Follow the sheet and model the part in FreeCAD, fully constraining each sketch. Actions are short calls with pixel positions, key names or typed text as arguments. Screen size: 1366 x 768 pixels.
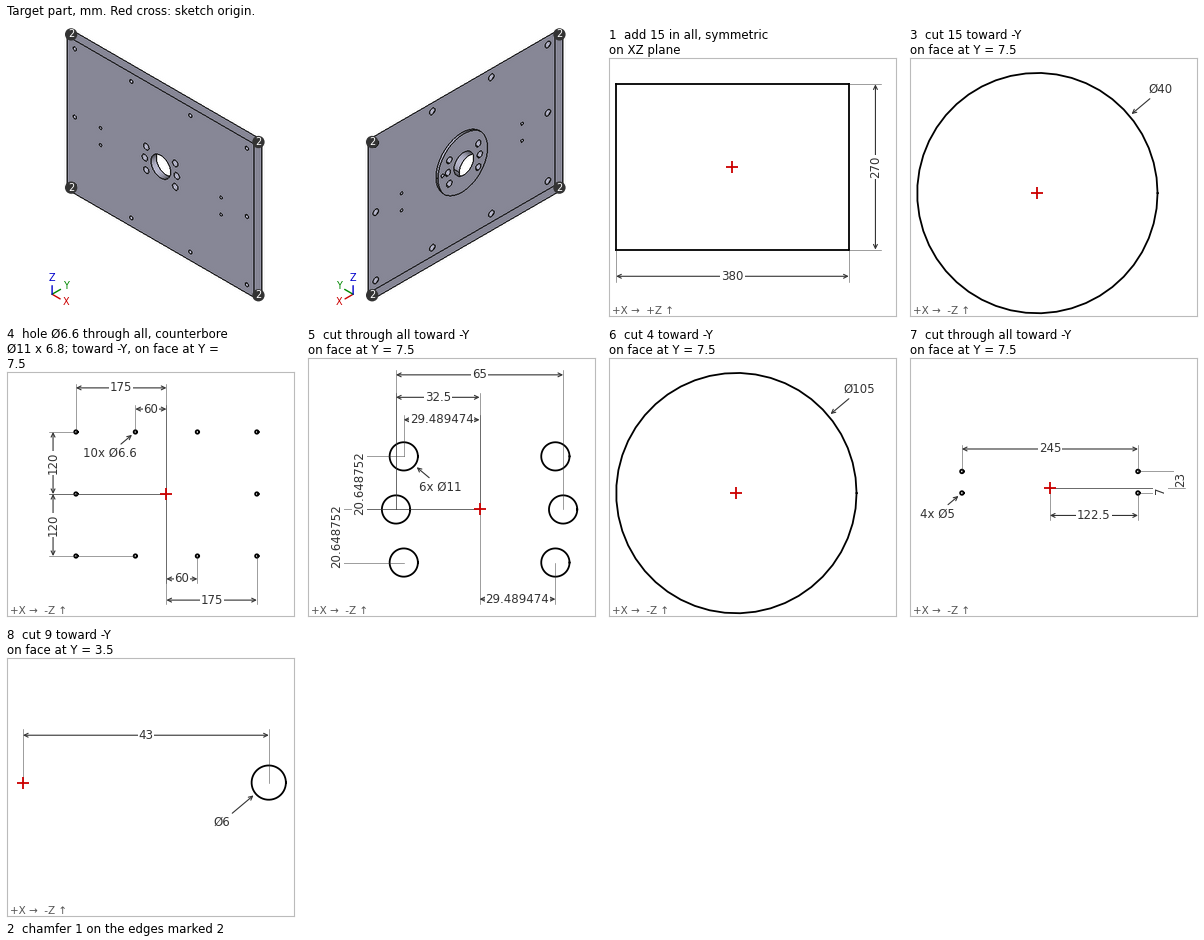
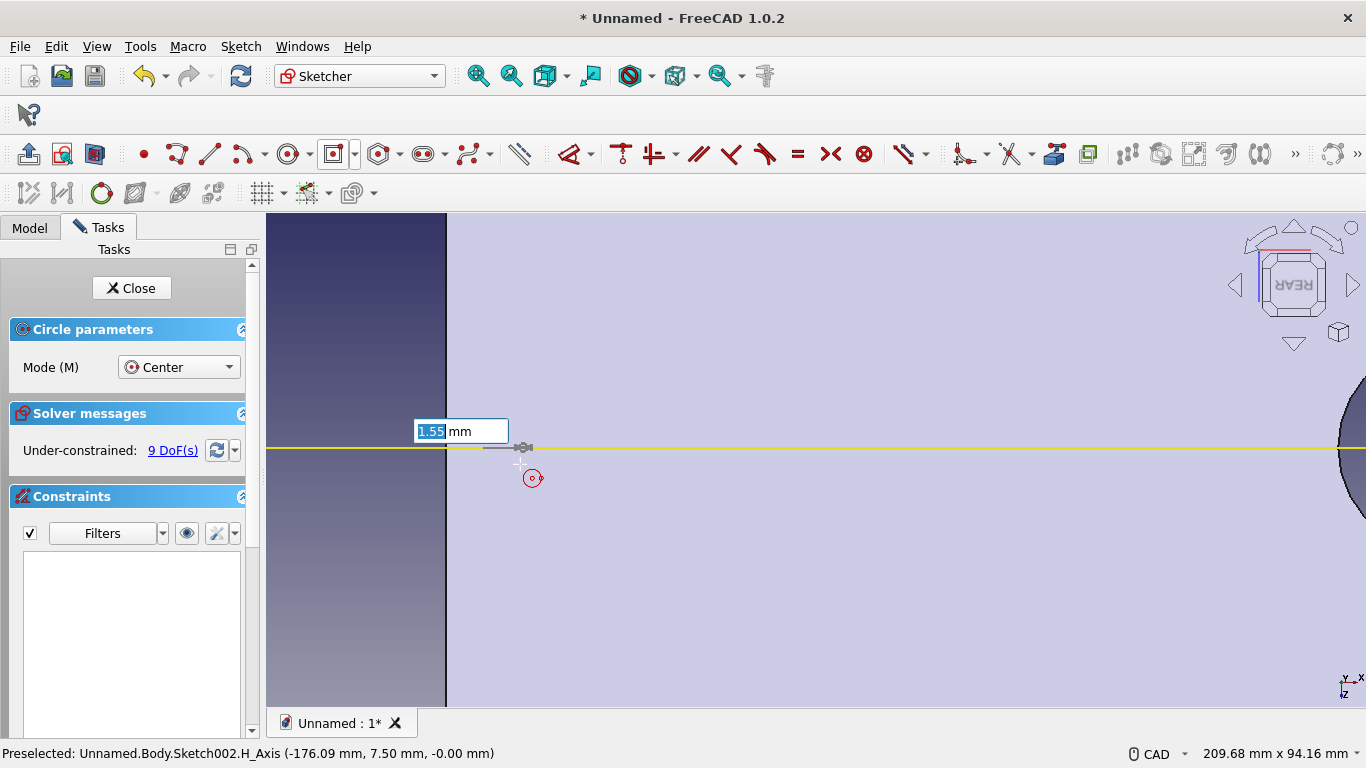
click(519, 464)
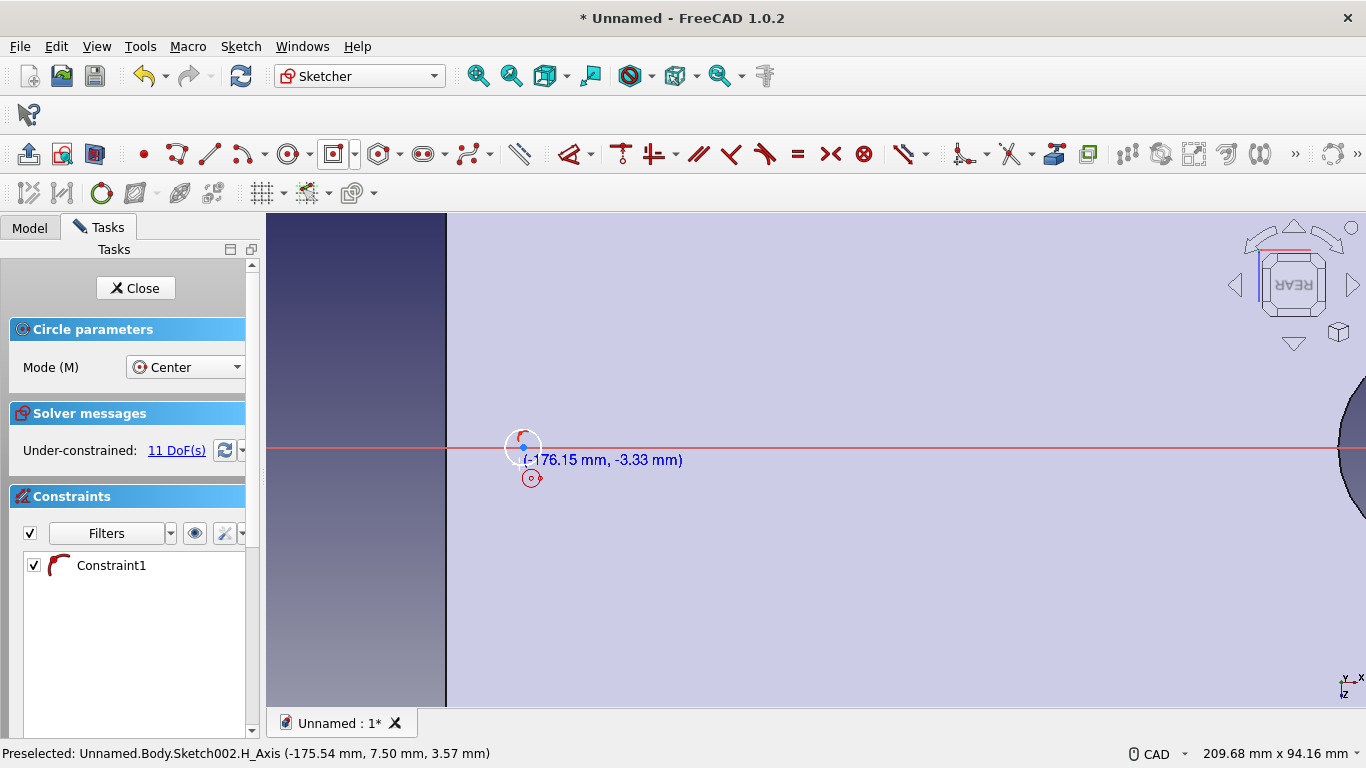
scroll(520, 464, down, 7)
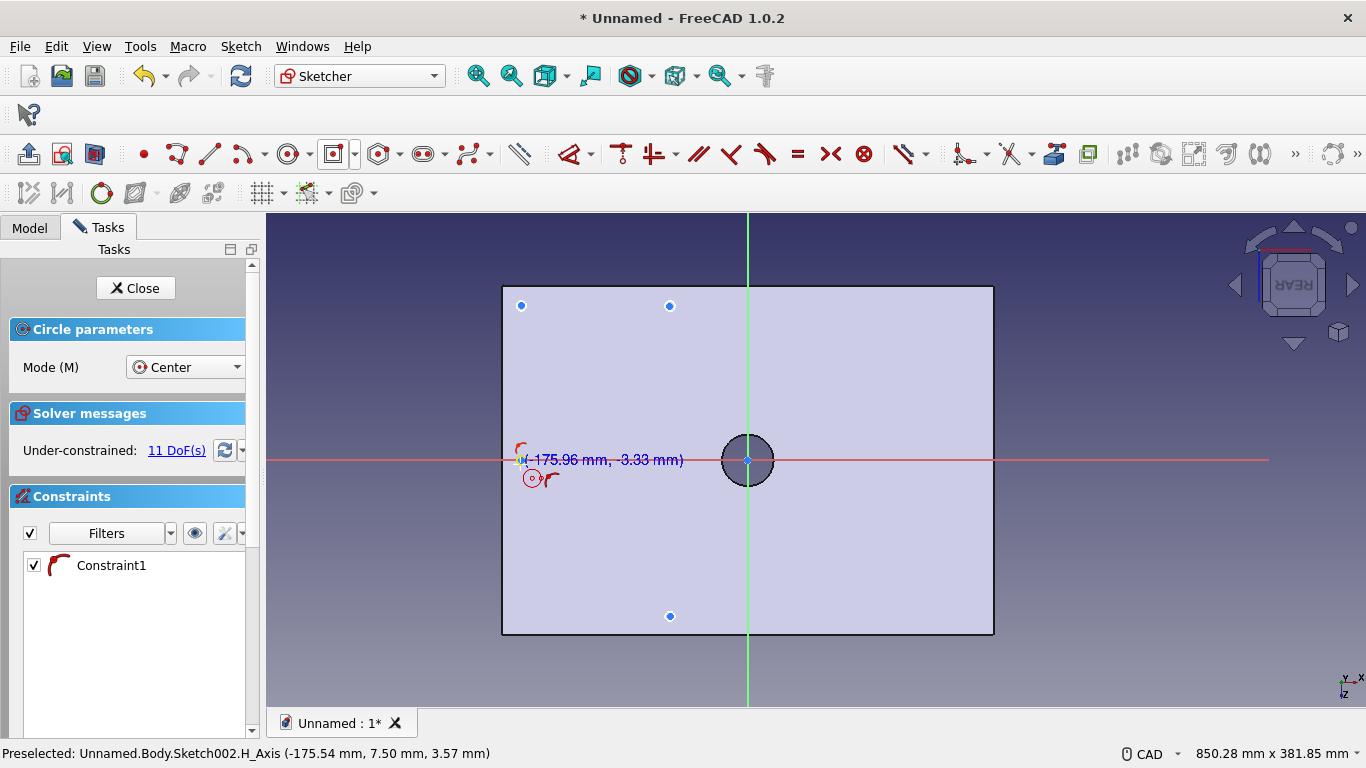
scroll(521, 616, up, 9)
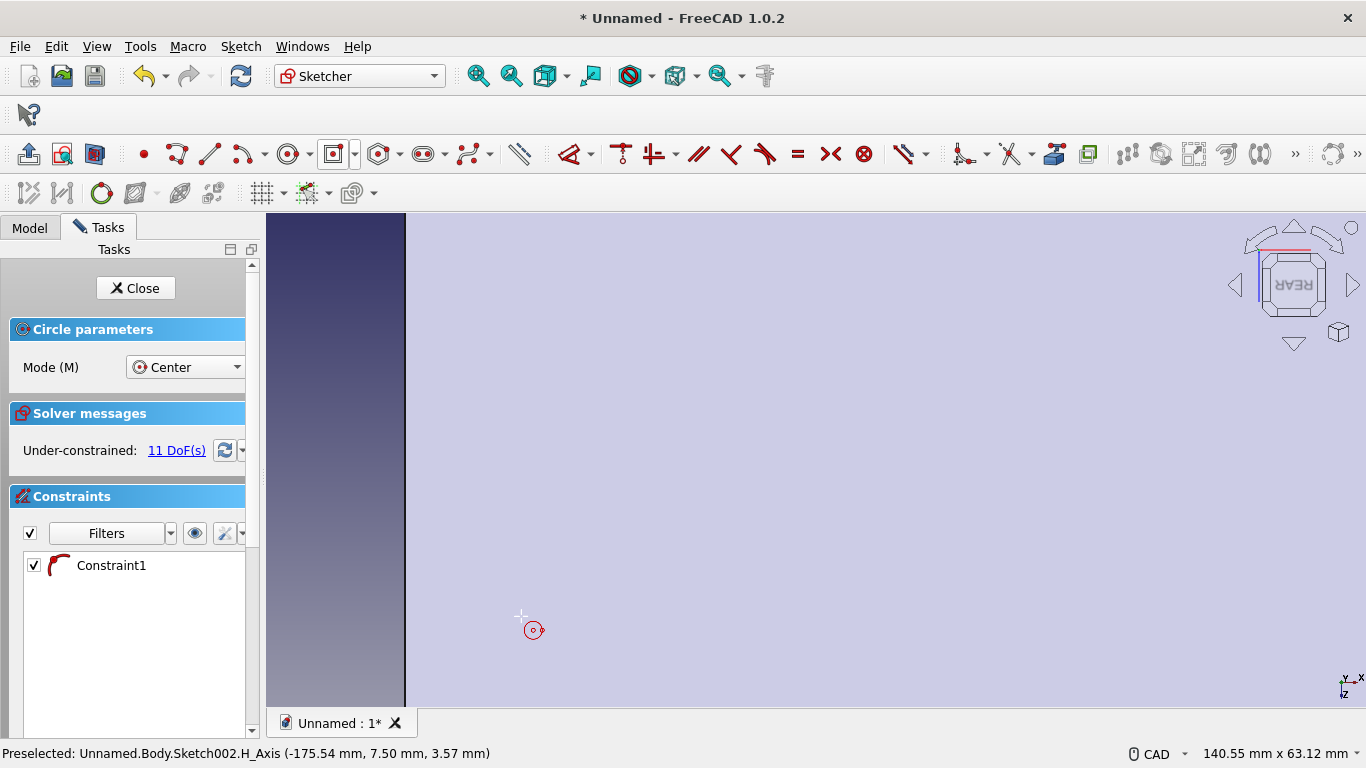
scroll(521, 616, down, 9)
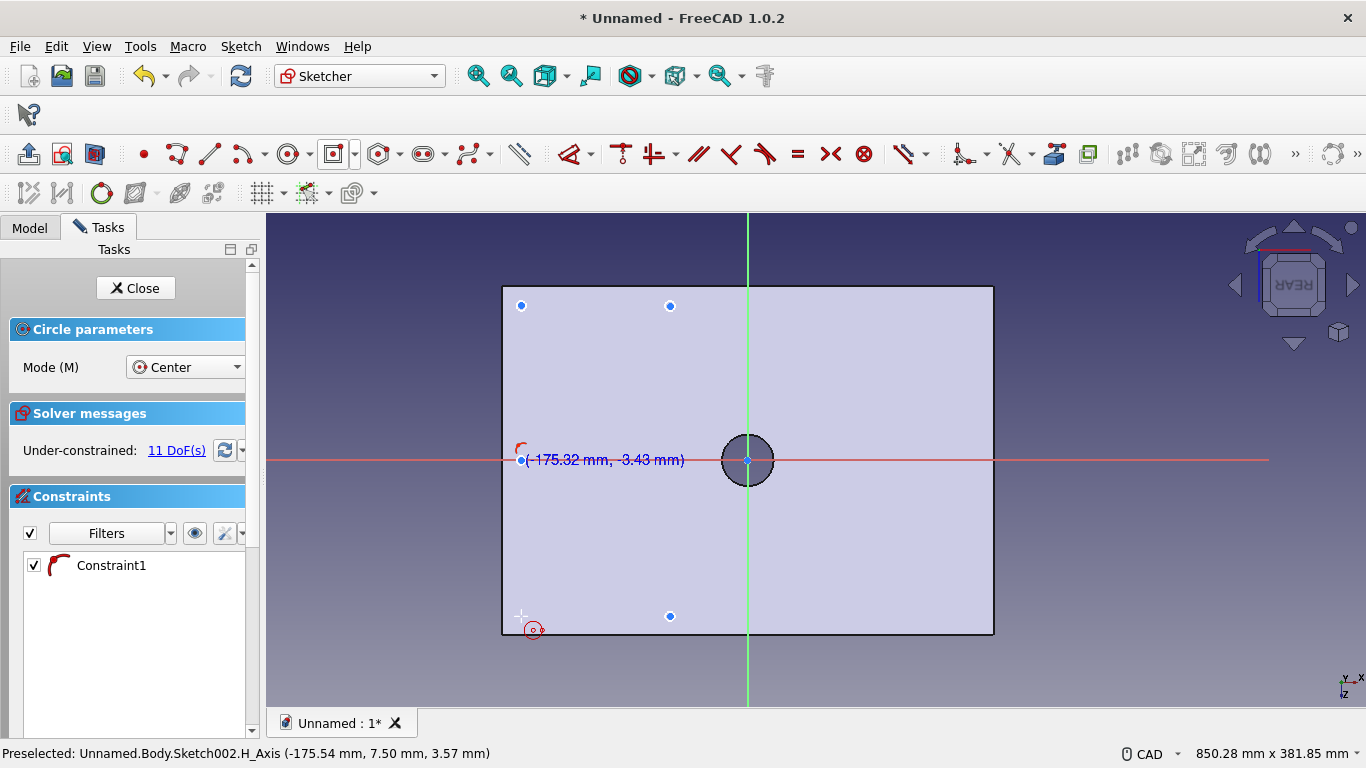
click(521, 616)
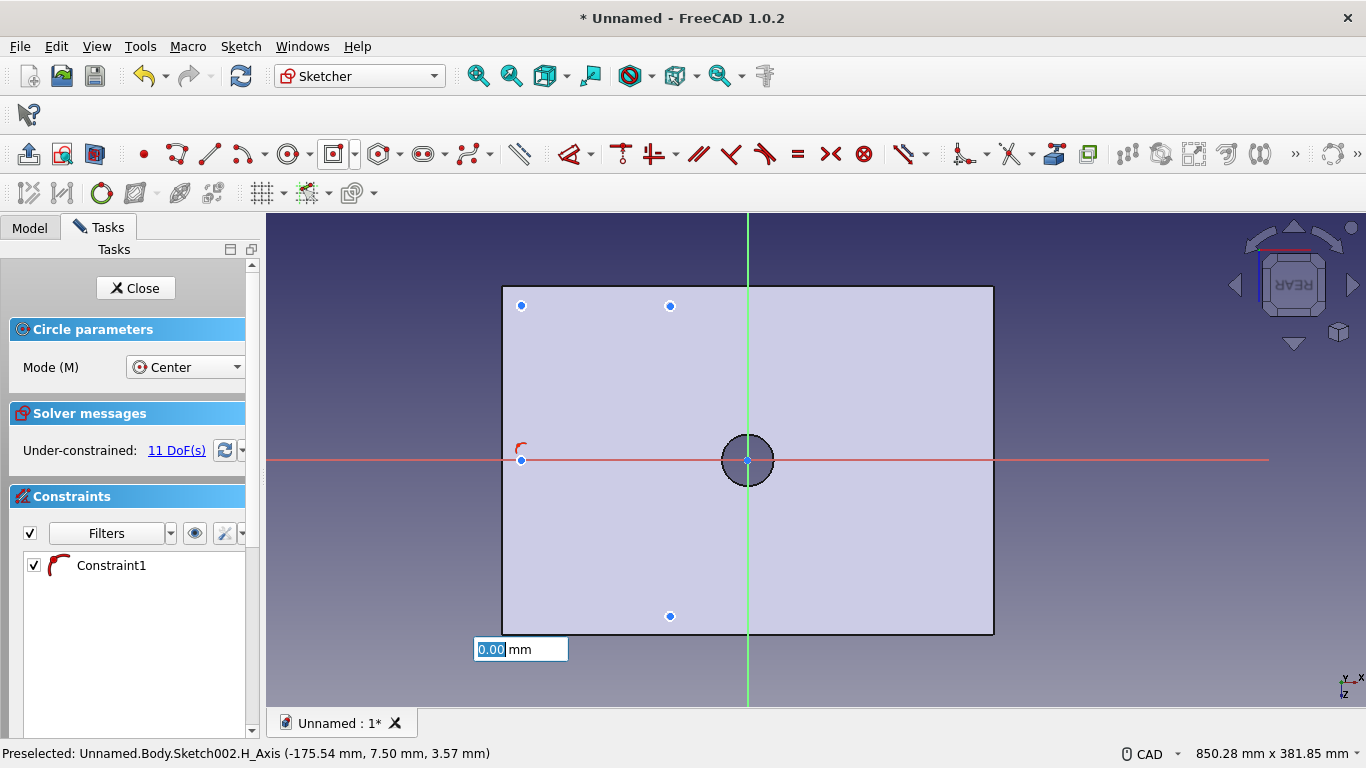
scroll(524, 613, up, 7)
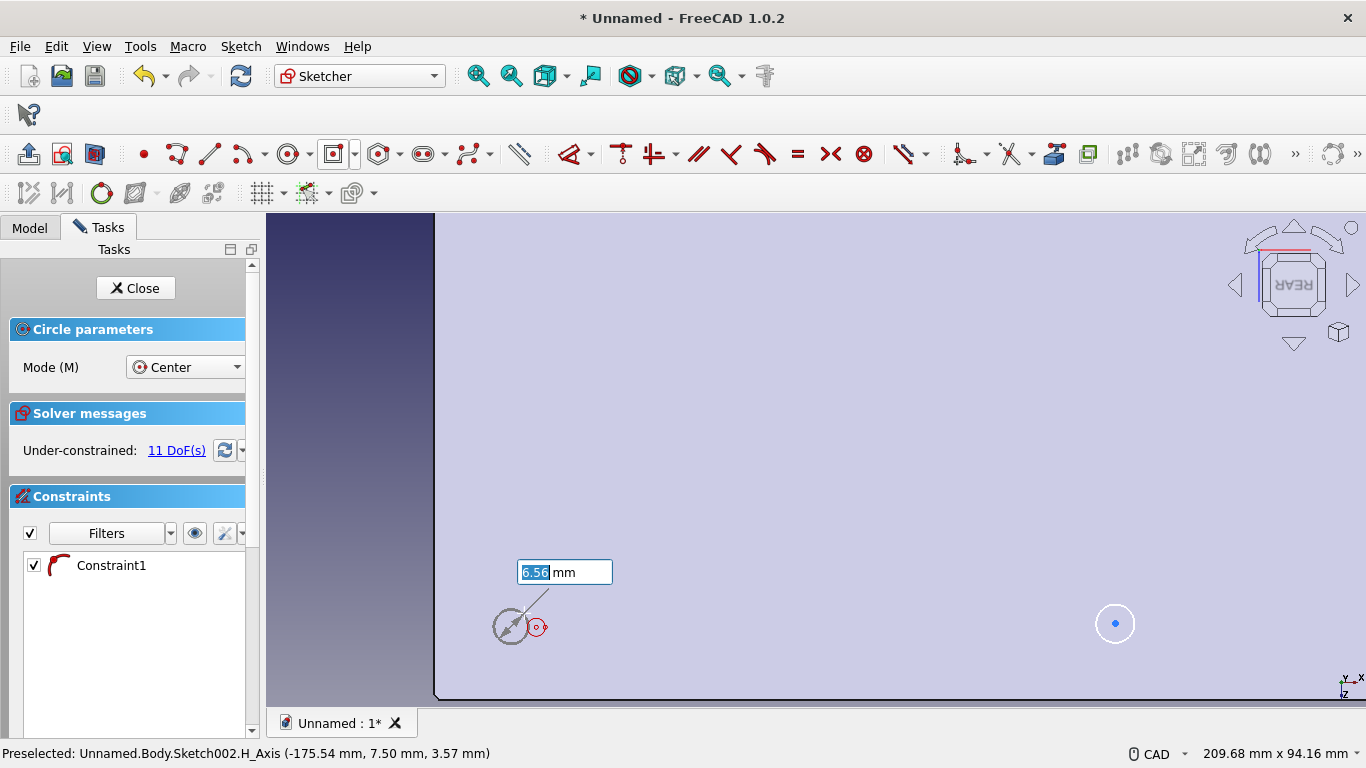
click(525, 609)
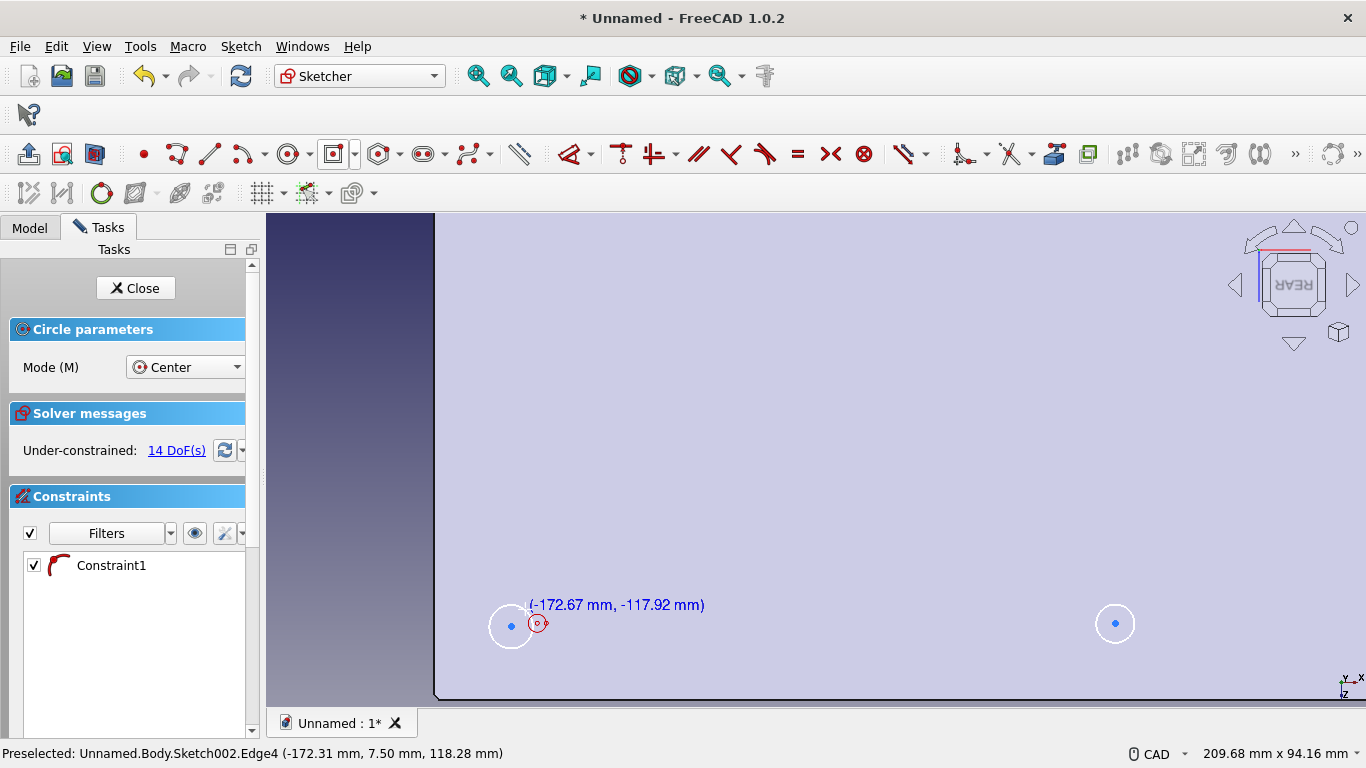
scroll(524, 613, down, 7)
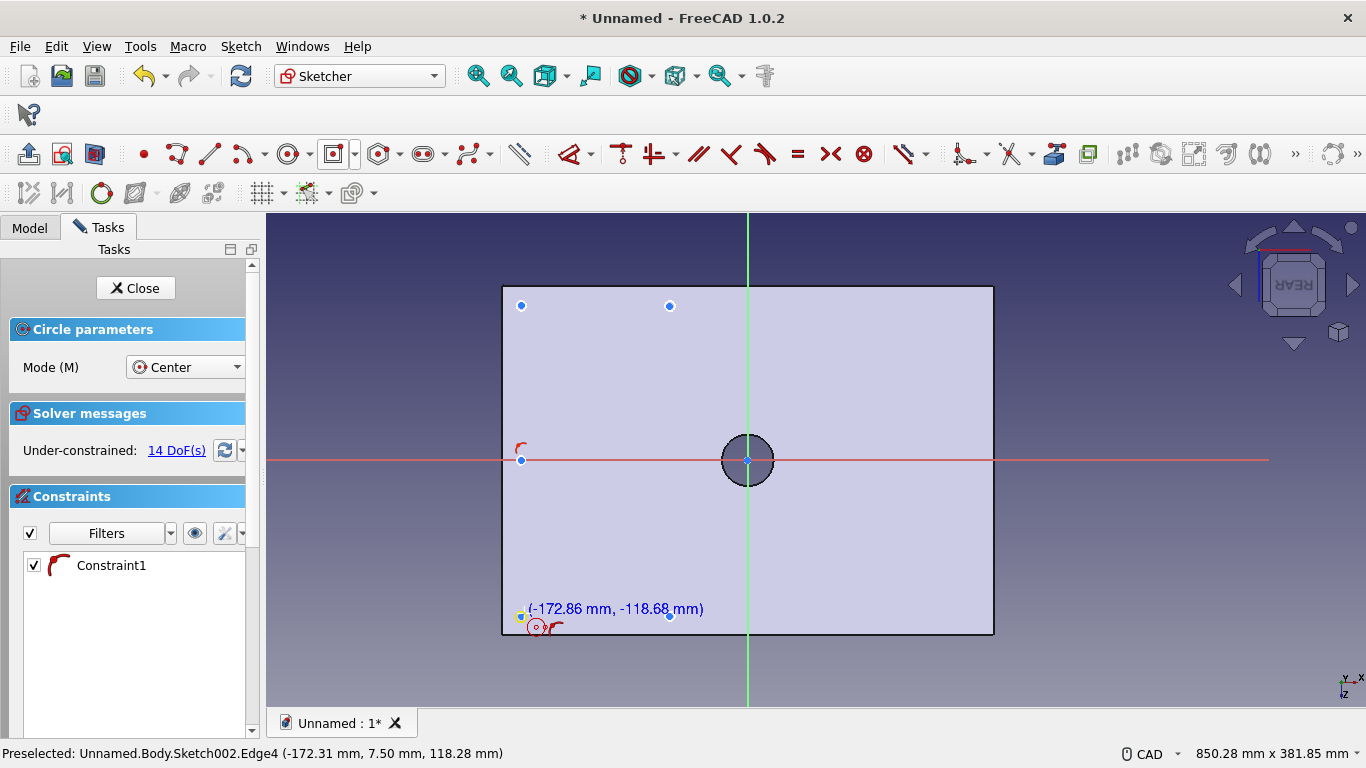
scroll(974, 616, up, 9)